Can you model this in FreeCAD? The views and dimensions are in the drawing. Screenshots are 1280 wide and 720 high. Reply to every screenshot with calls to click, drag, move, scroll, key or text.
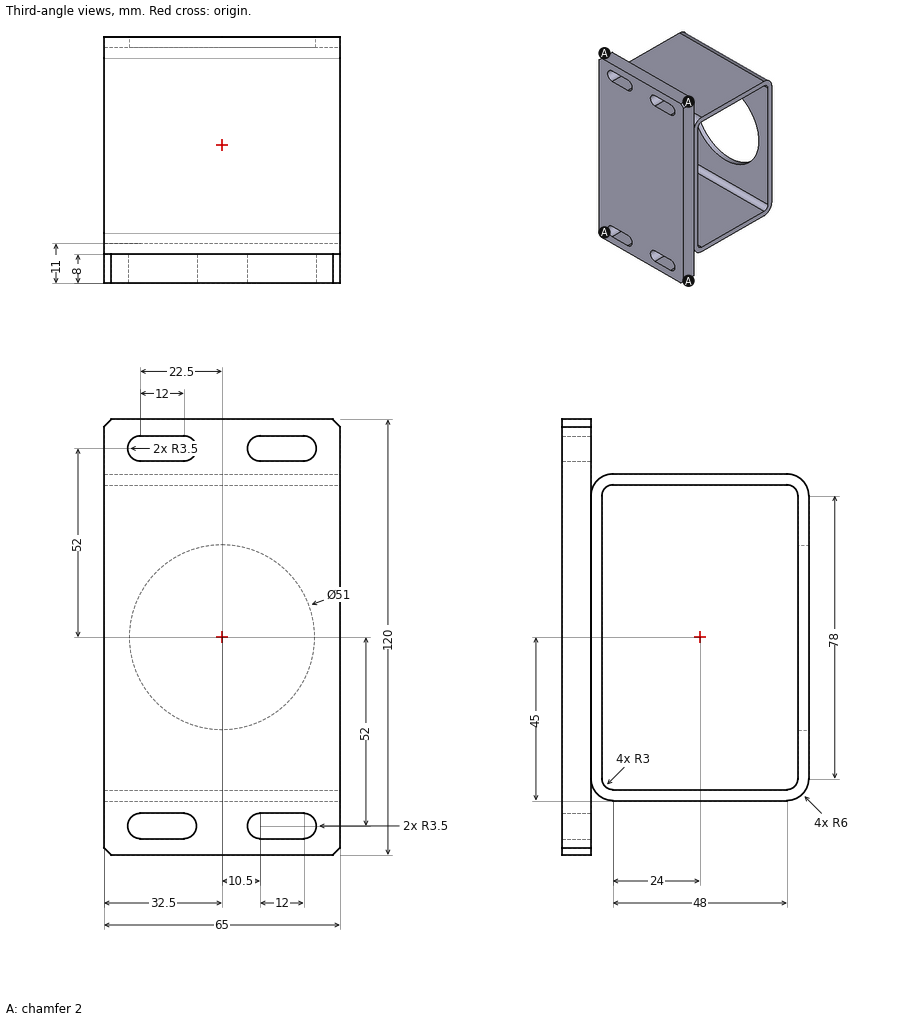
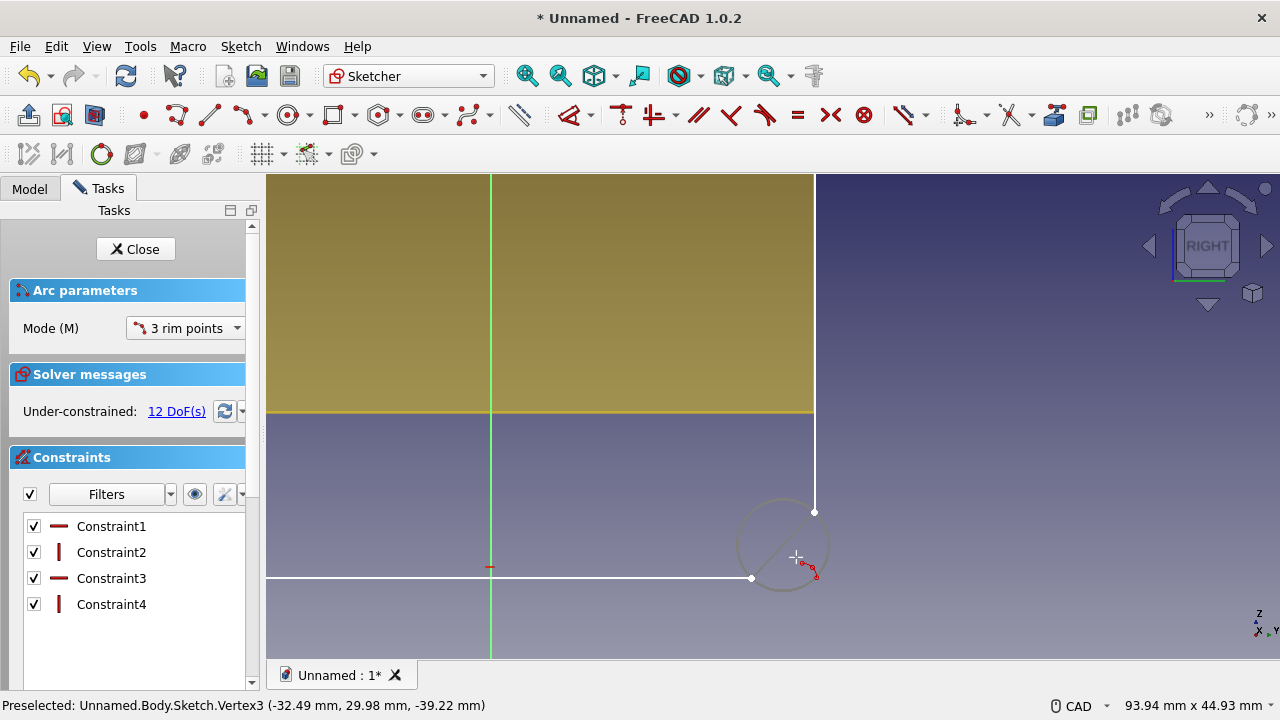
click(796, 555)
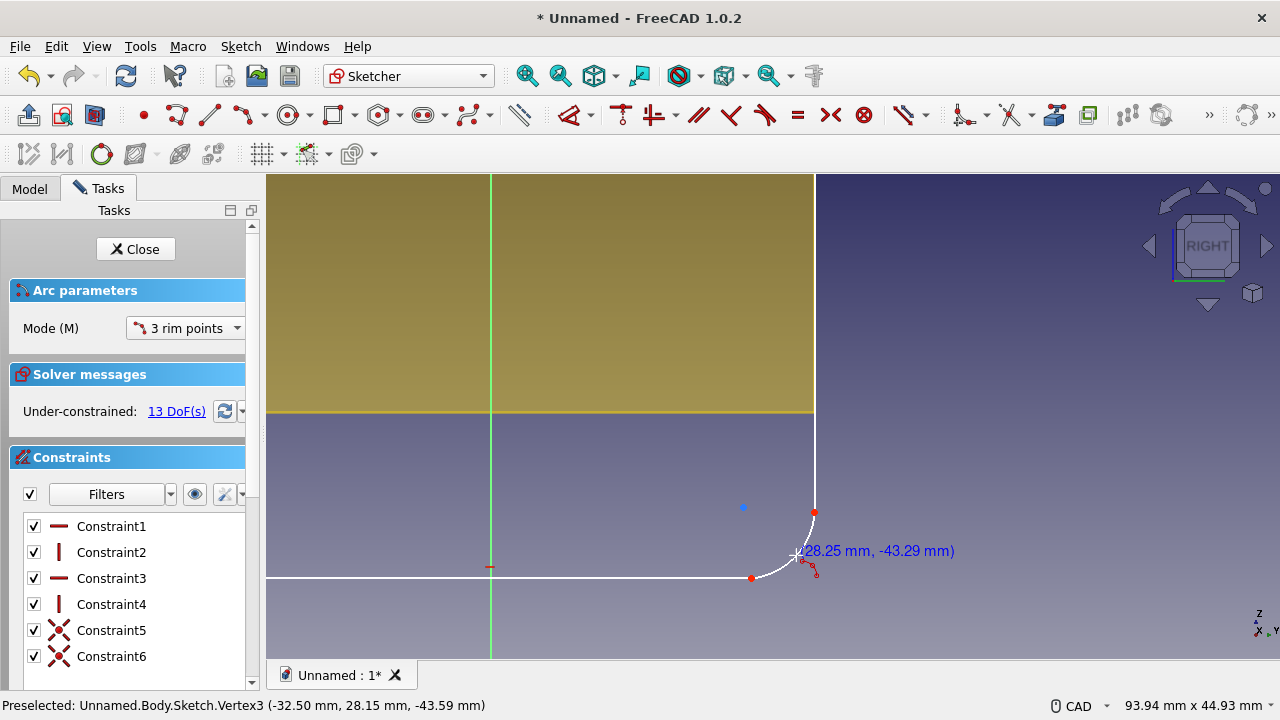
scroll(796, 558, down, 6)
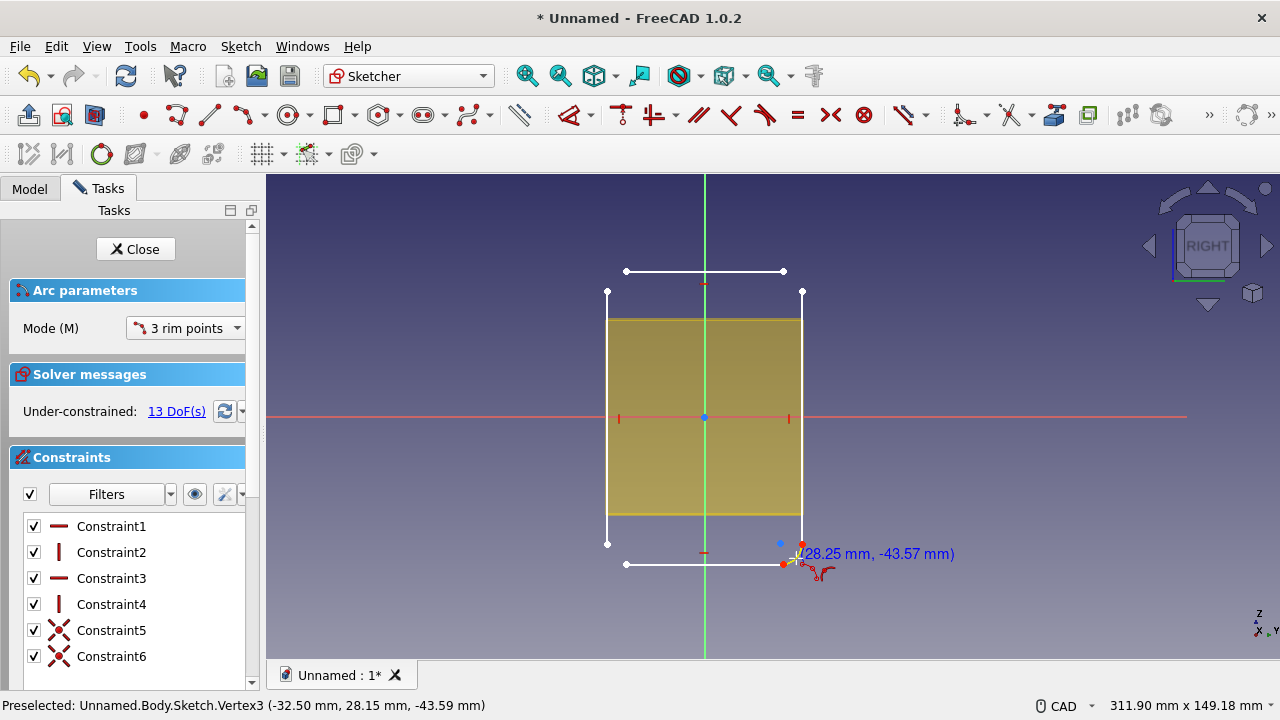
click(802, 292)
click(783, 272)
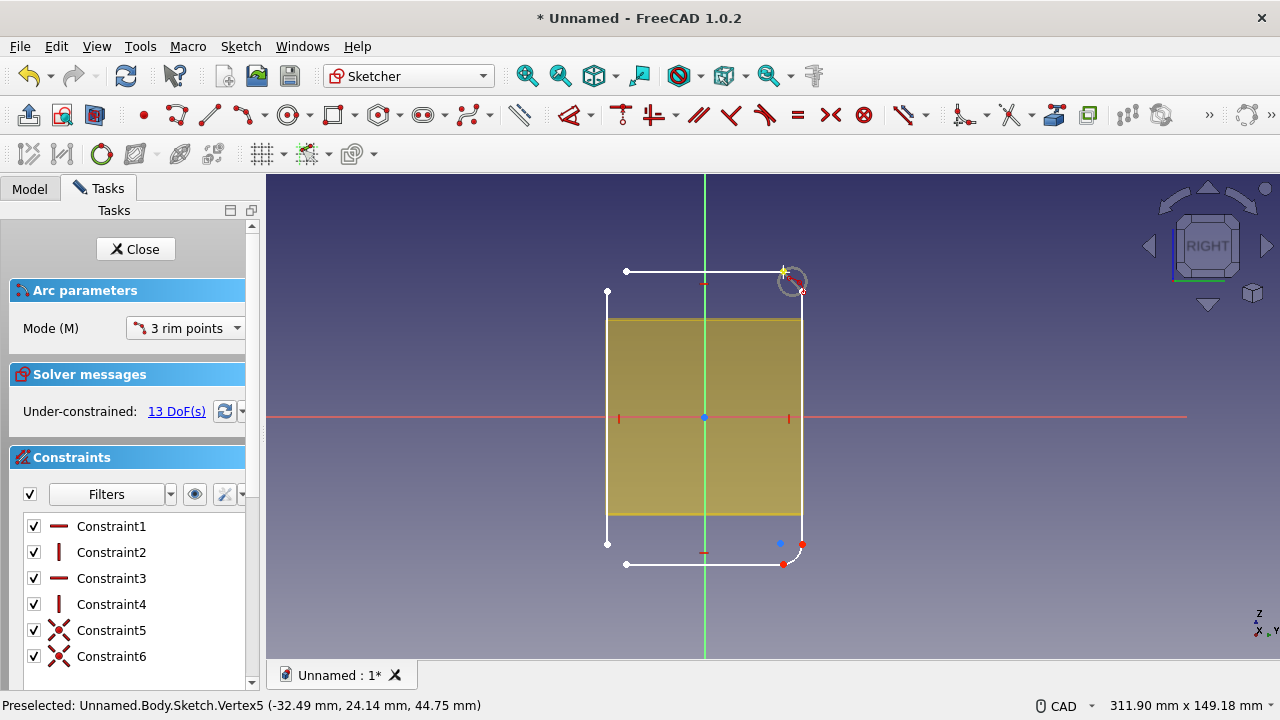
scroll(796, 277, up, 6)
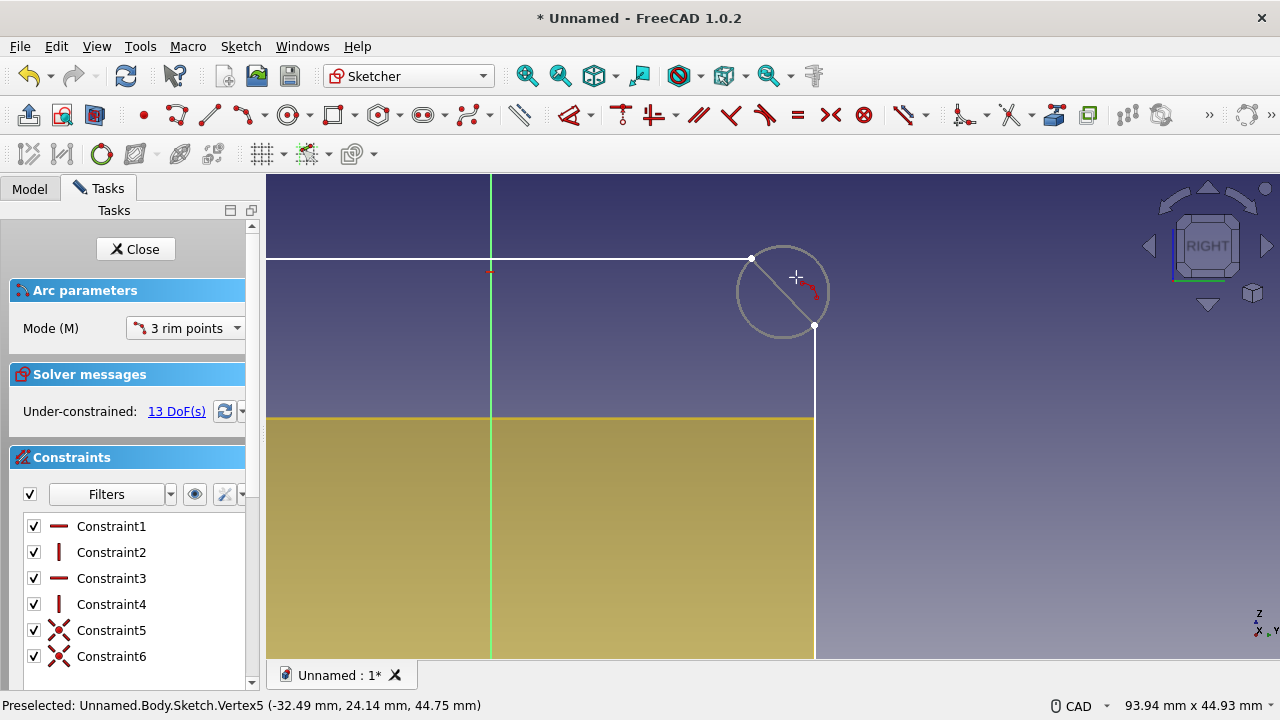
click(796, 275)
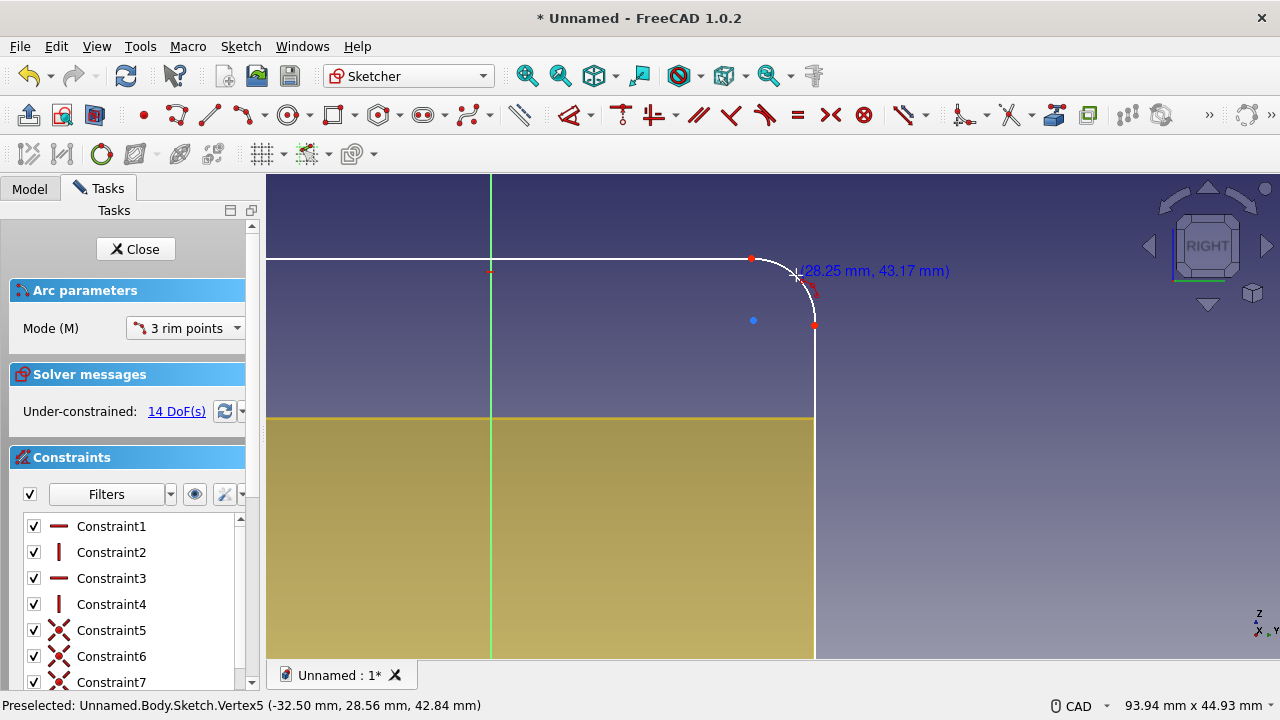
scroll(796, 276, down, 6)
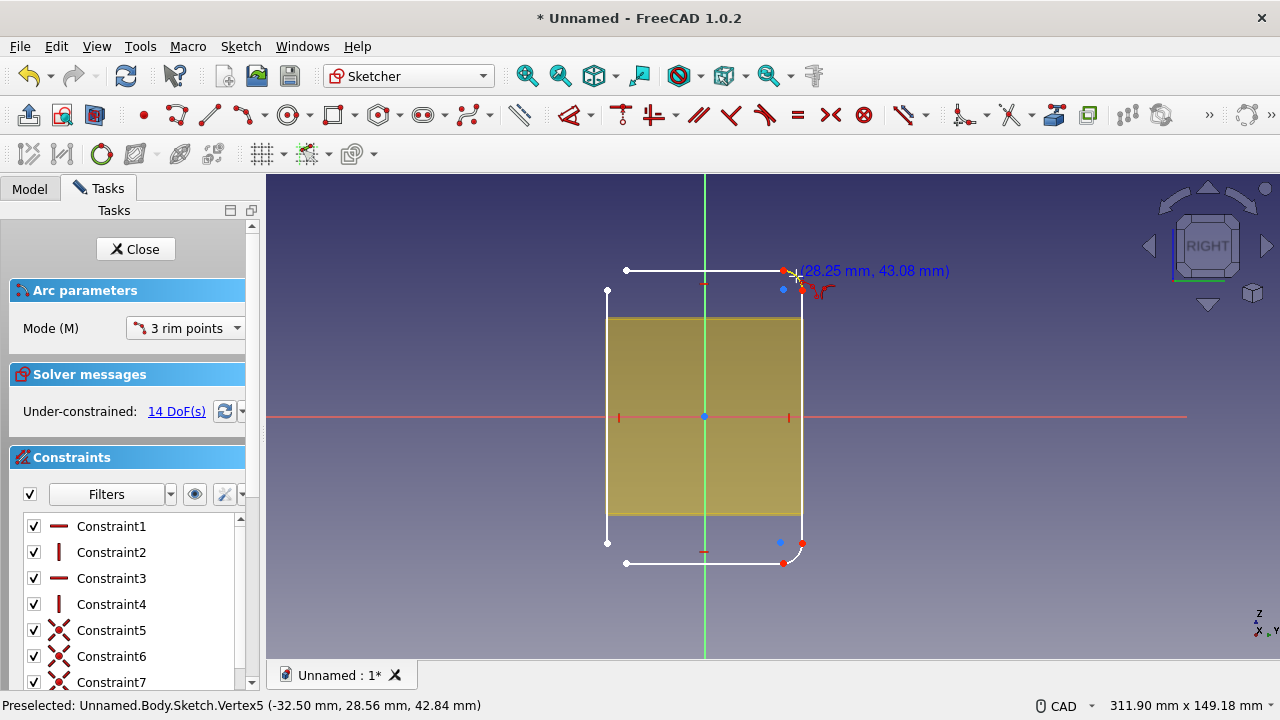
click(626, 271)
click(607, 291)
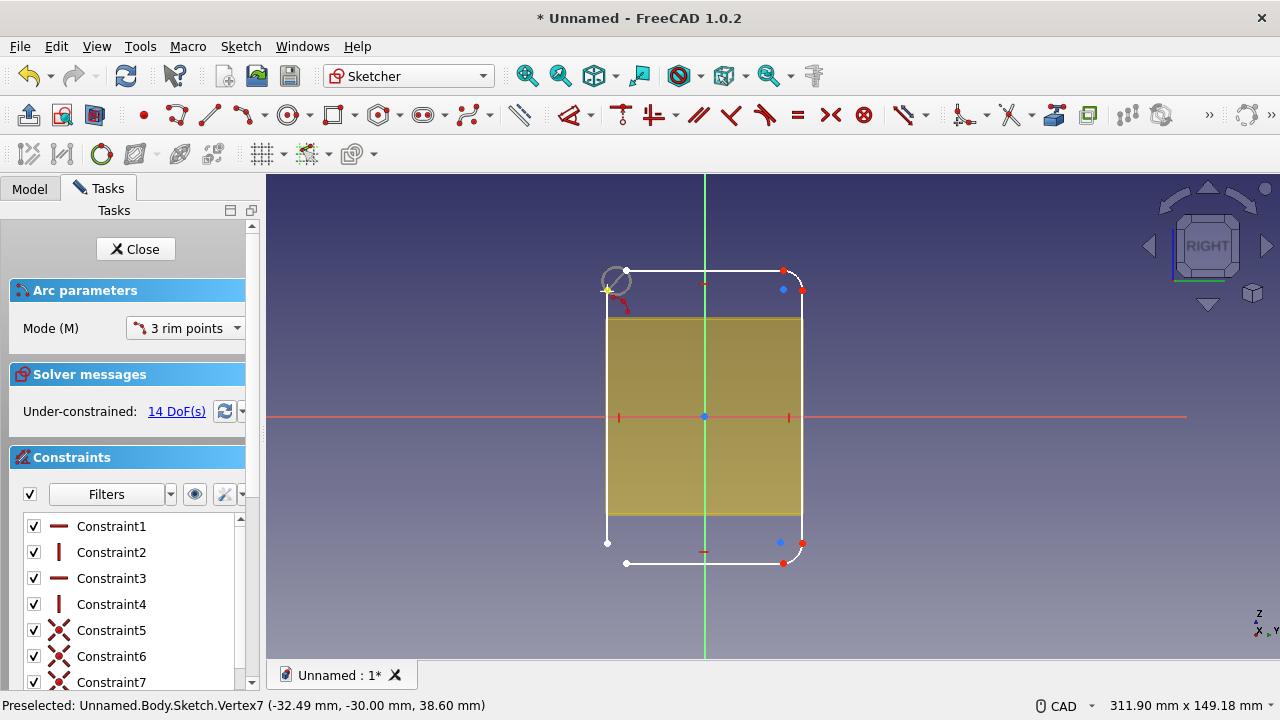
scroll(613, 276, up, 6)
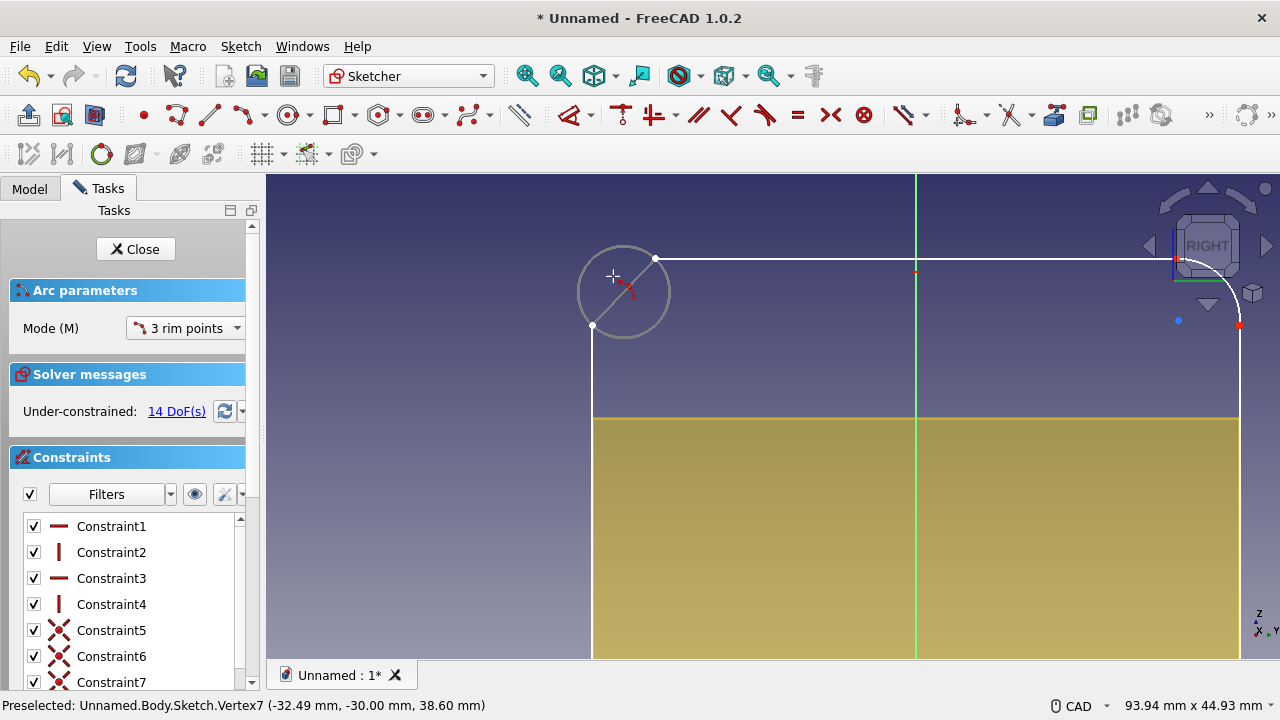
click(611, 275)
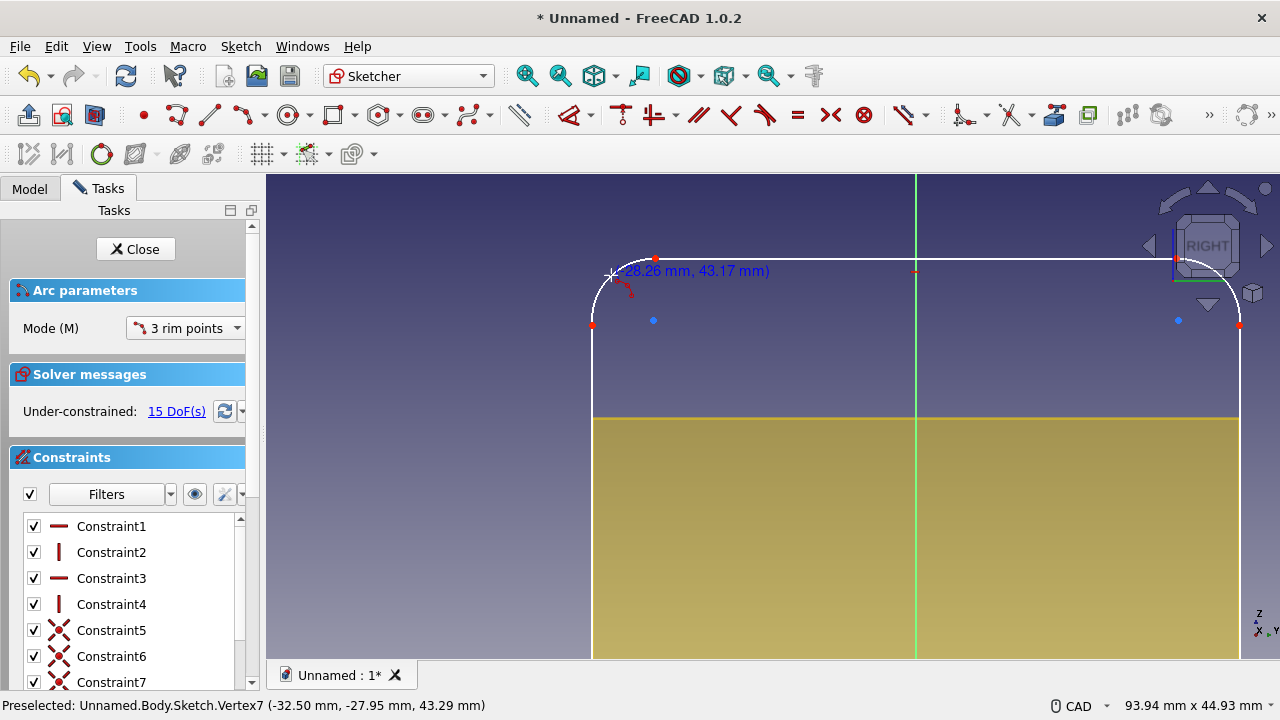
scroll(613, 276, down, 6)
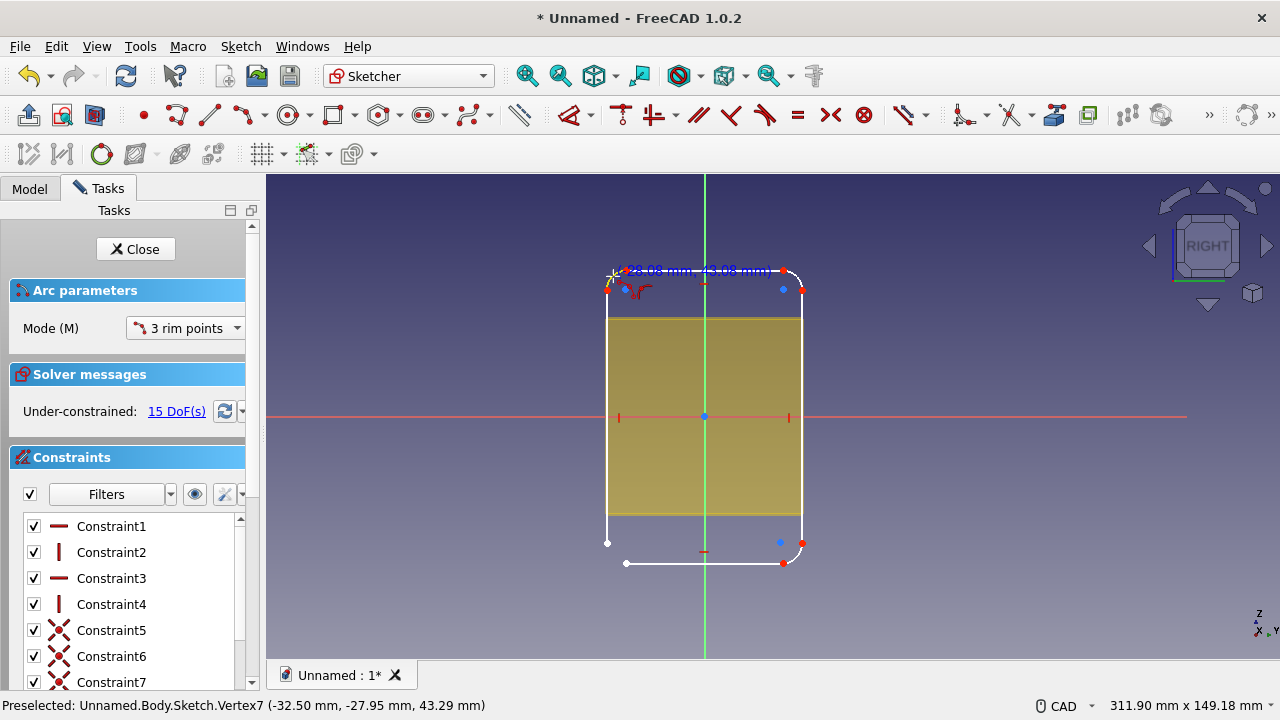
click(607, 544)
click(626, 564)